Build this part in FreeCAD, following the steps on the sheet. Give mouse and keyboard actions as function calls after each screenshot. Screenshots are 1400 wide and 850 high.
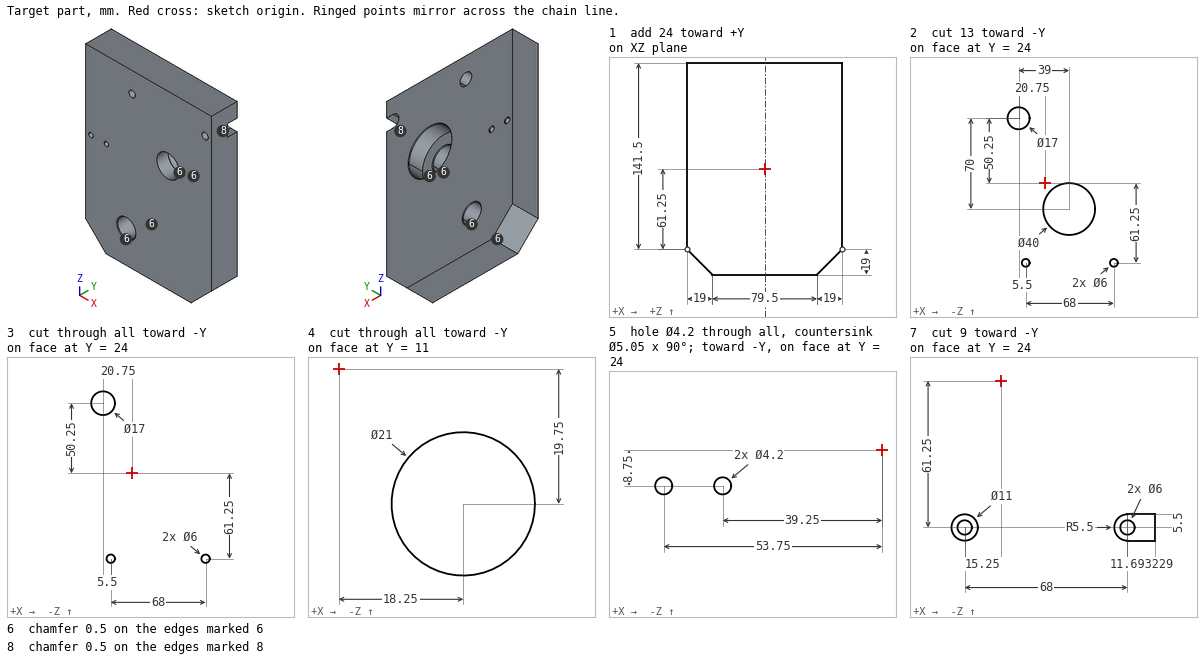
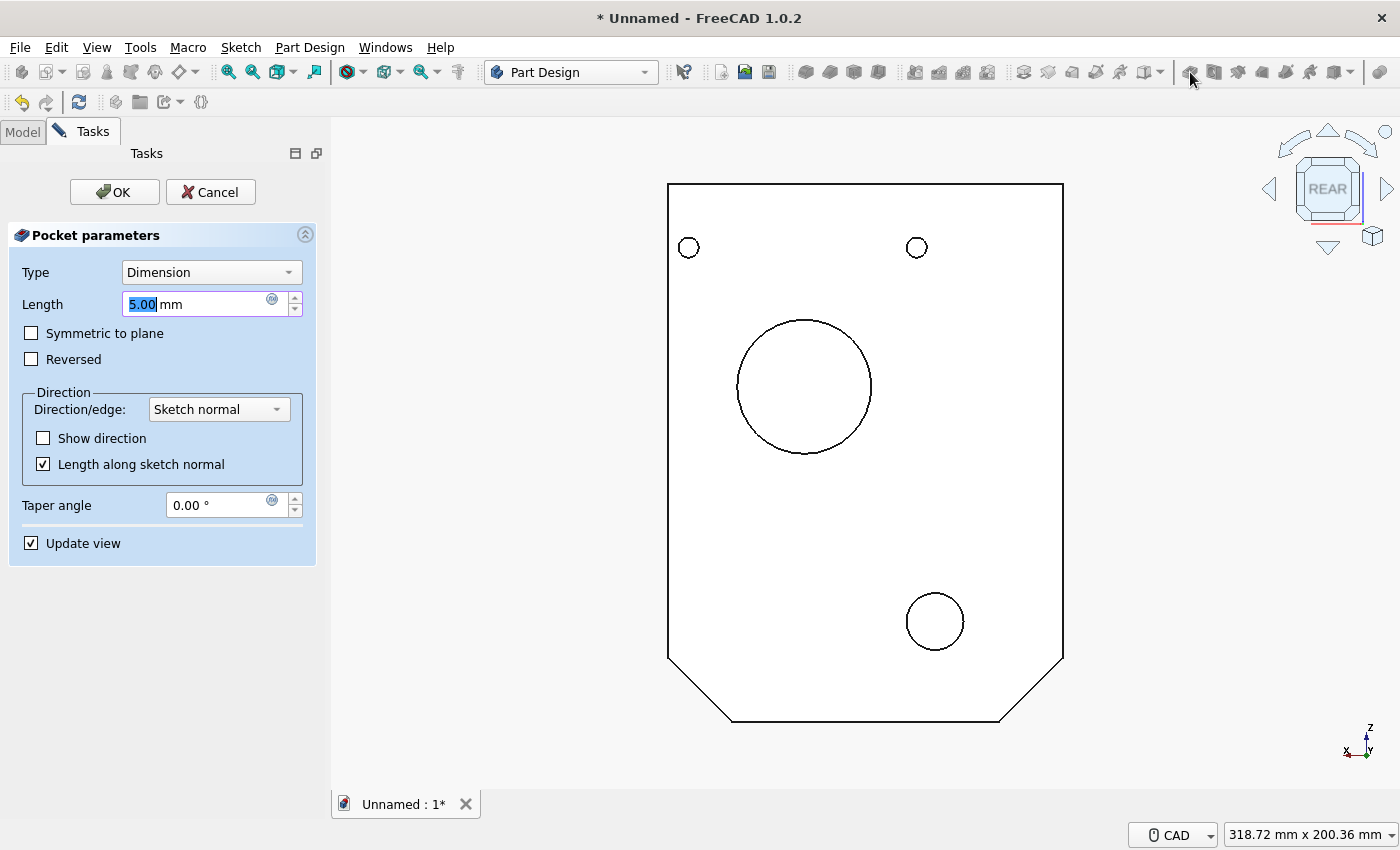
text(13)
key(Tab)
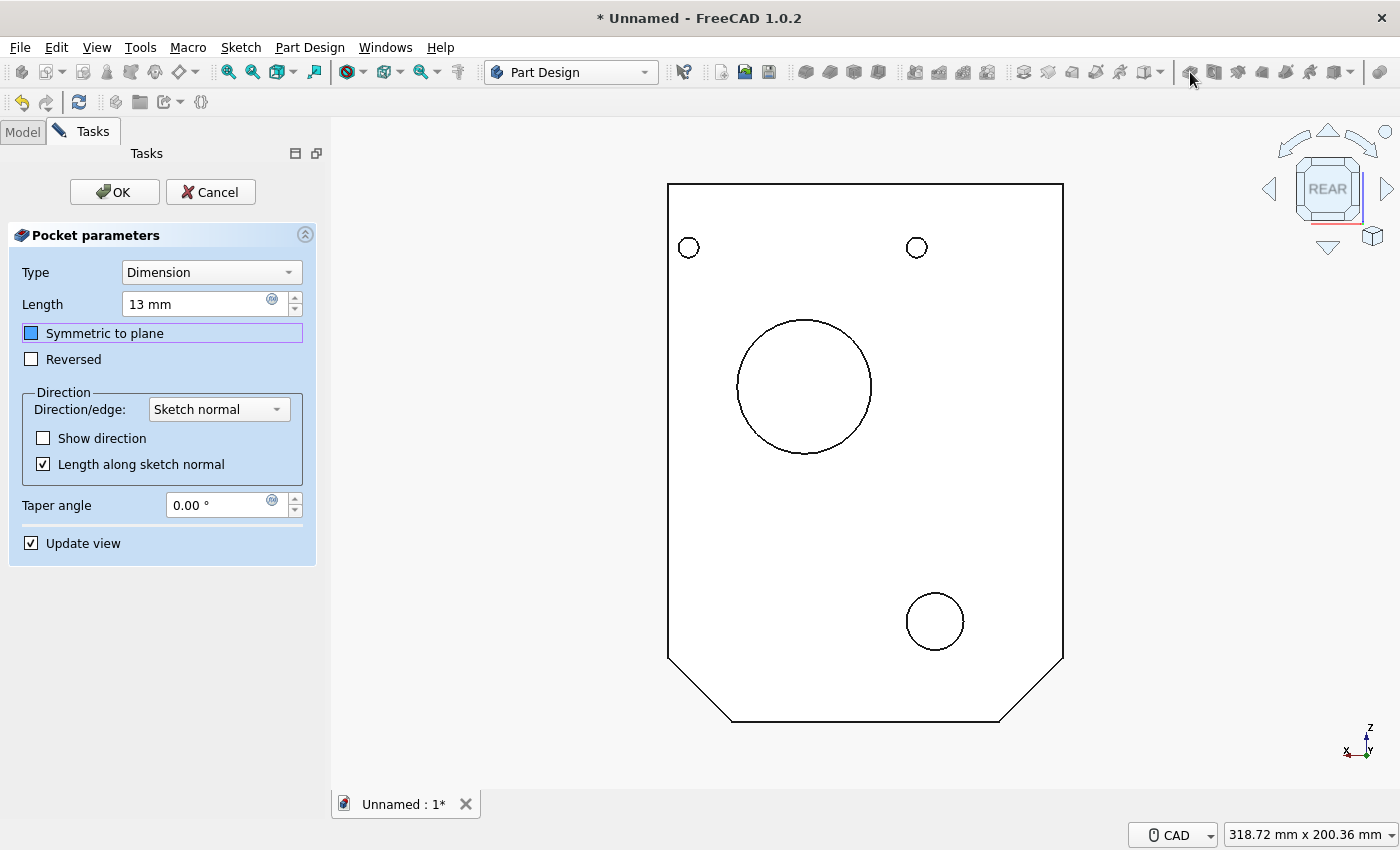
click(115, 192)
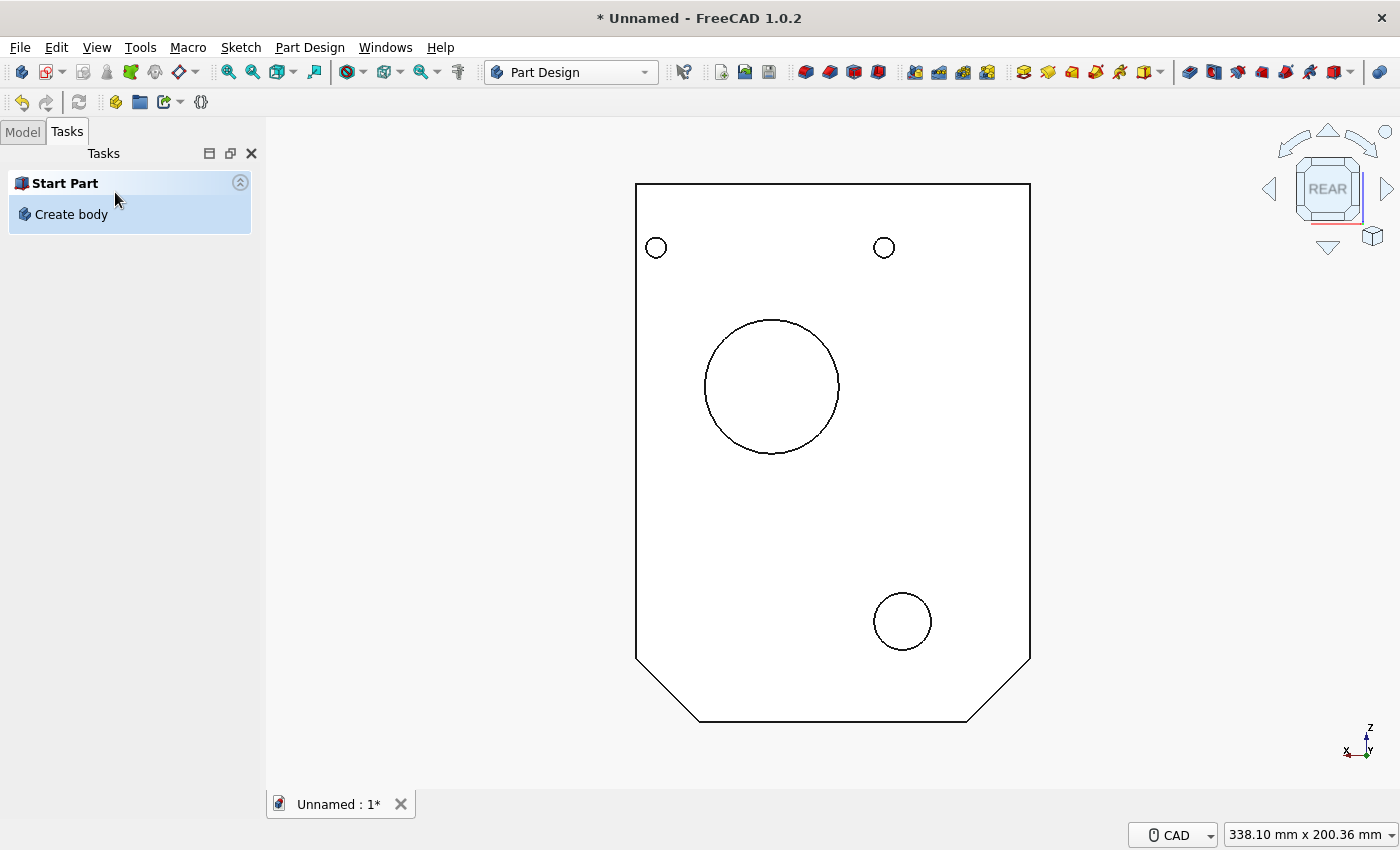
click(777, 606)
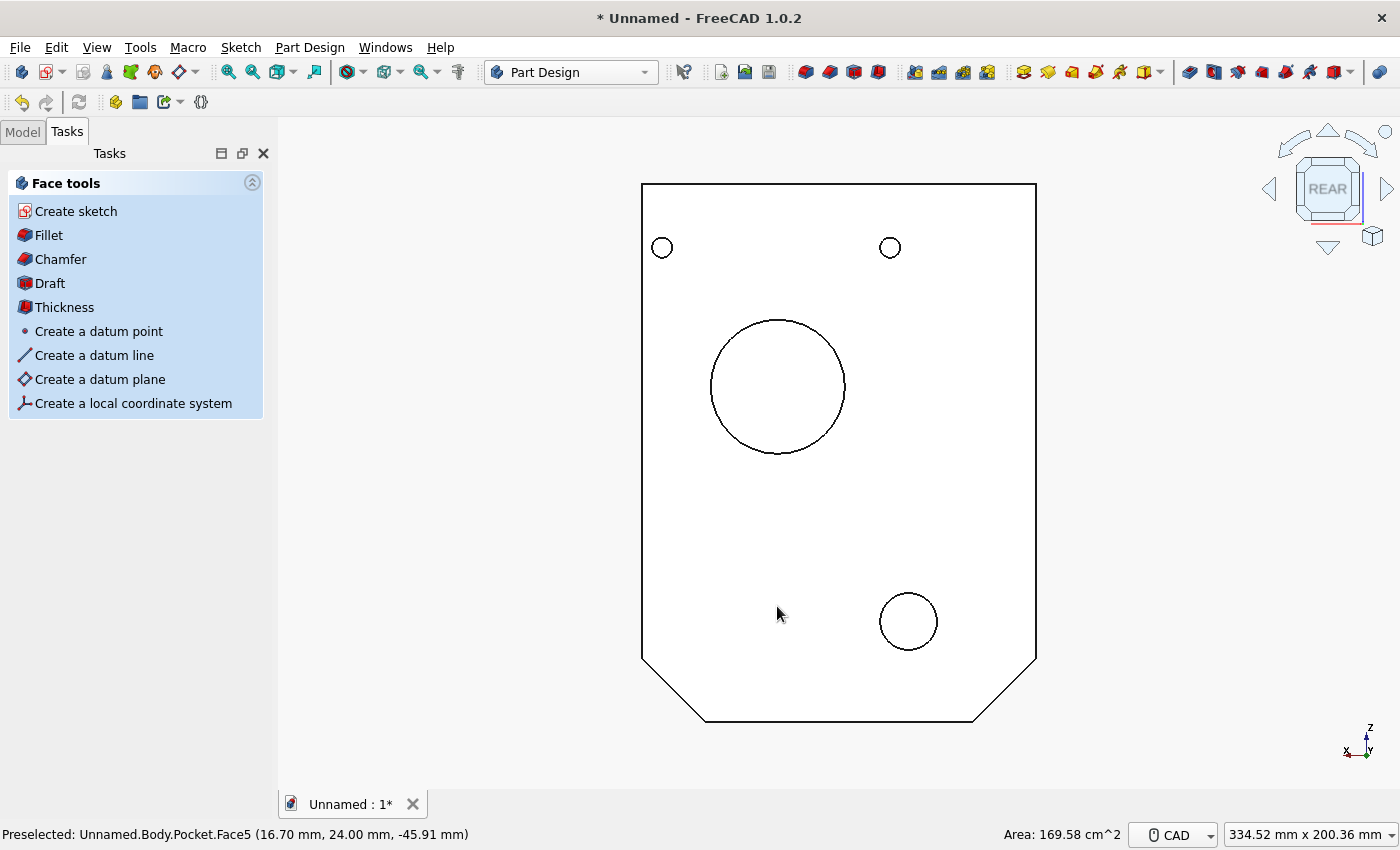
click(46, 72)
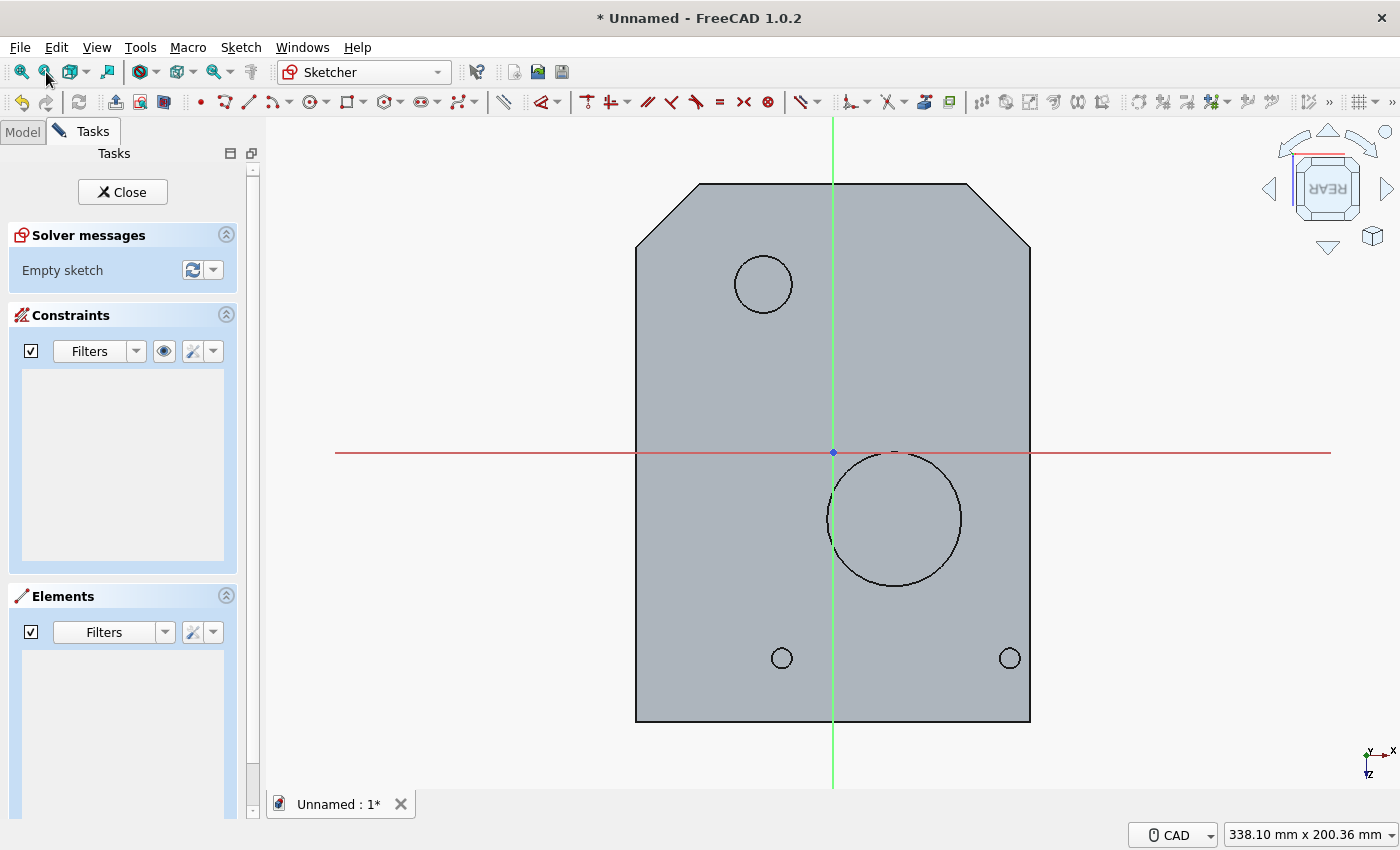
click(310, 102)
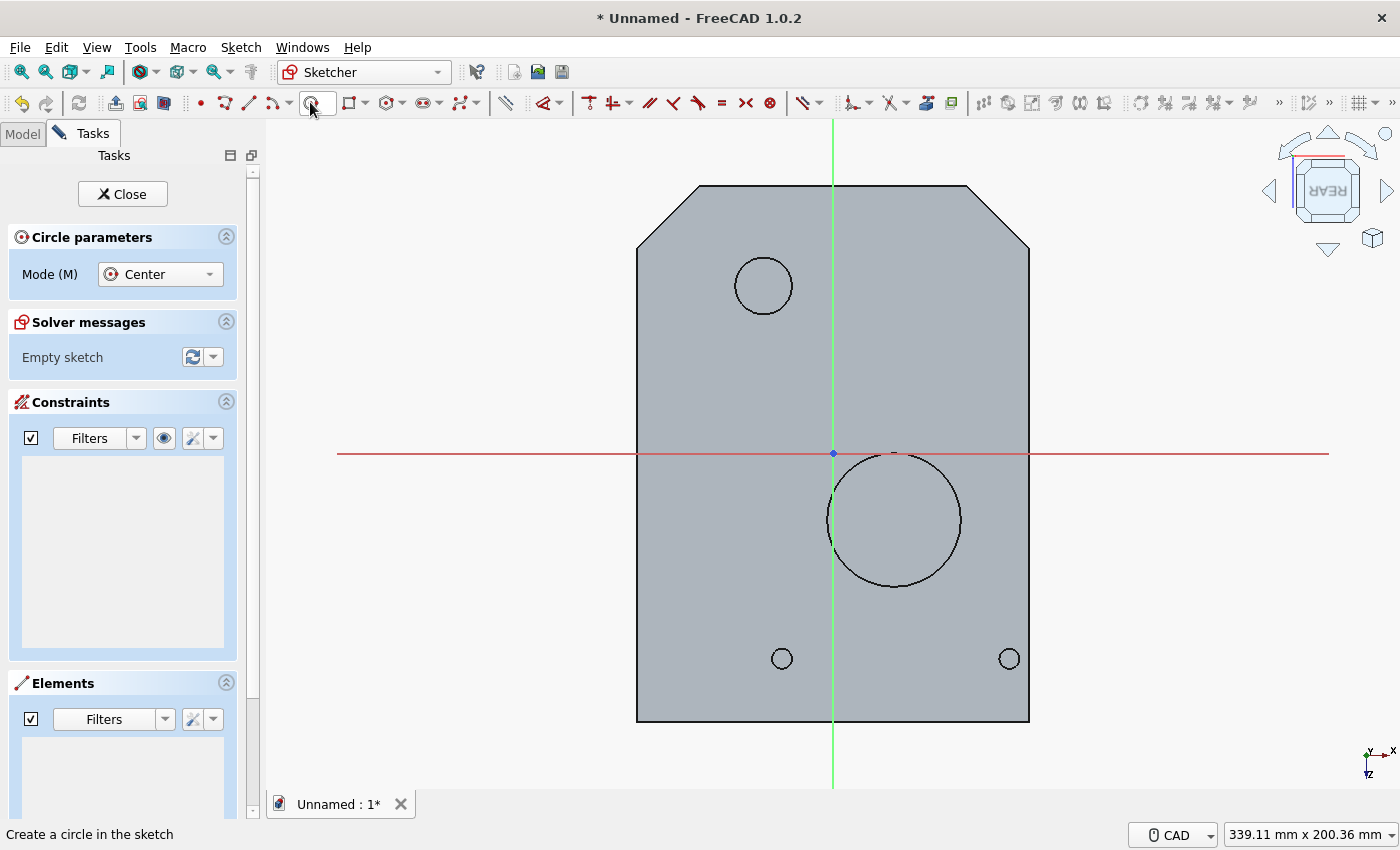
click(764, 286)
move(784, 266)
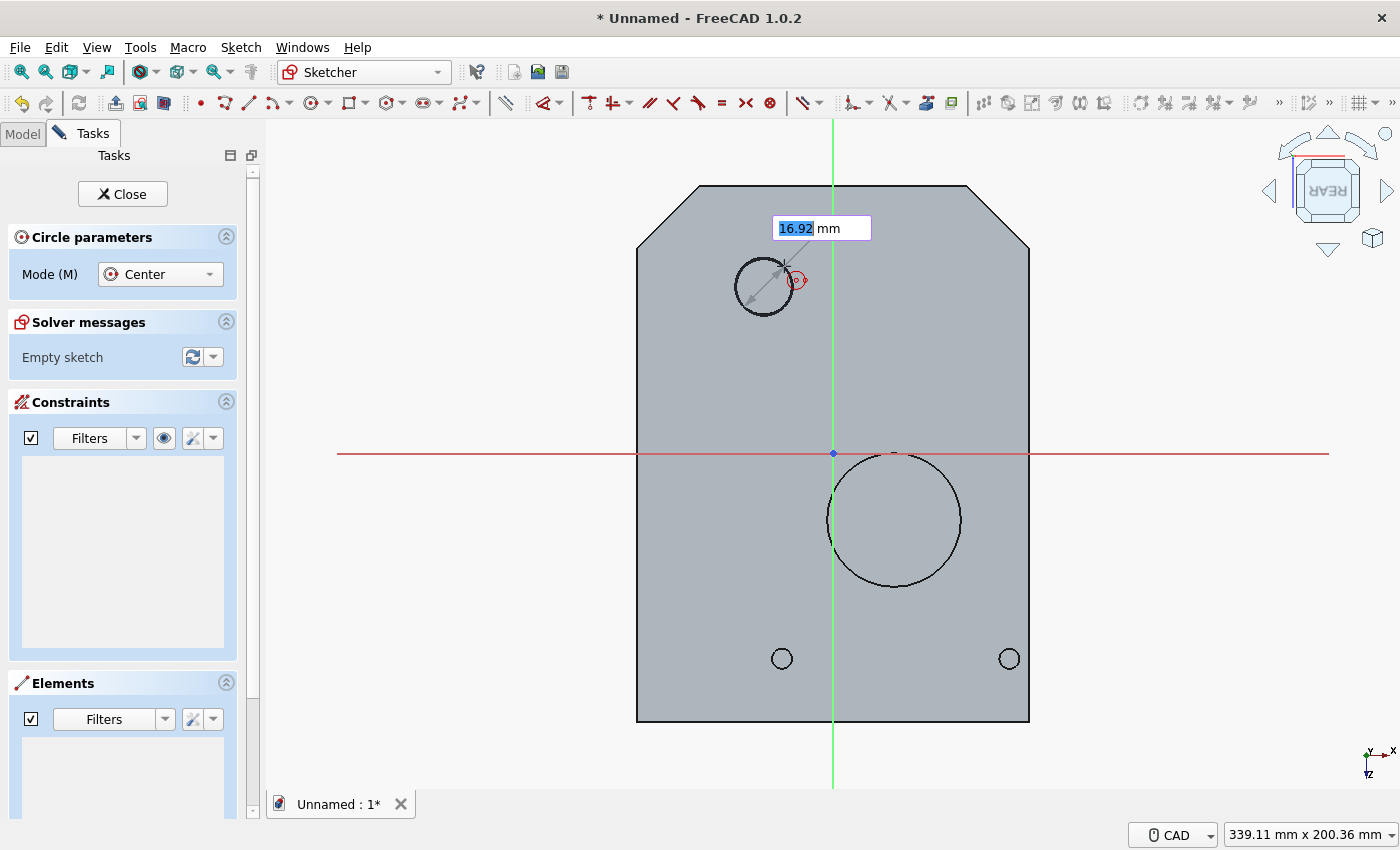
text(17)
key(Return)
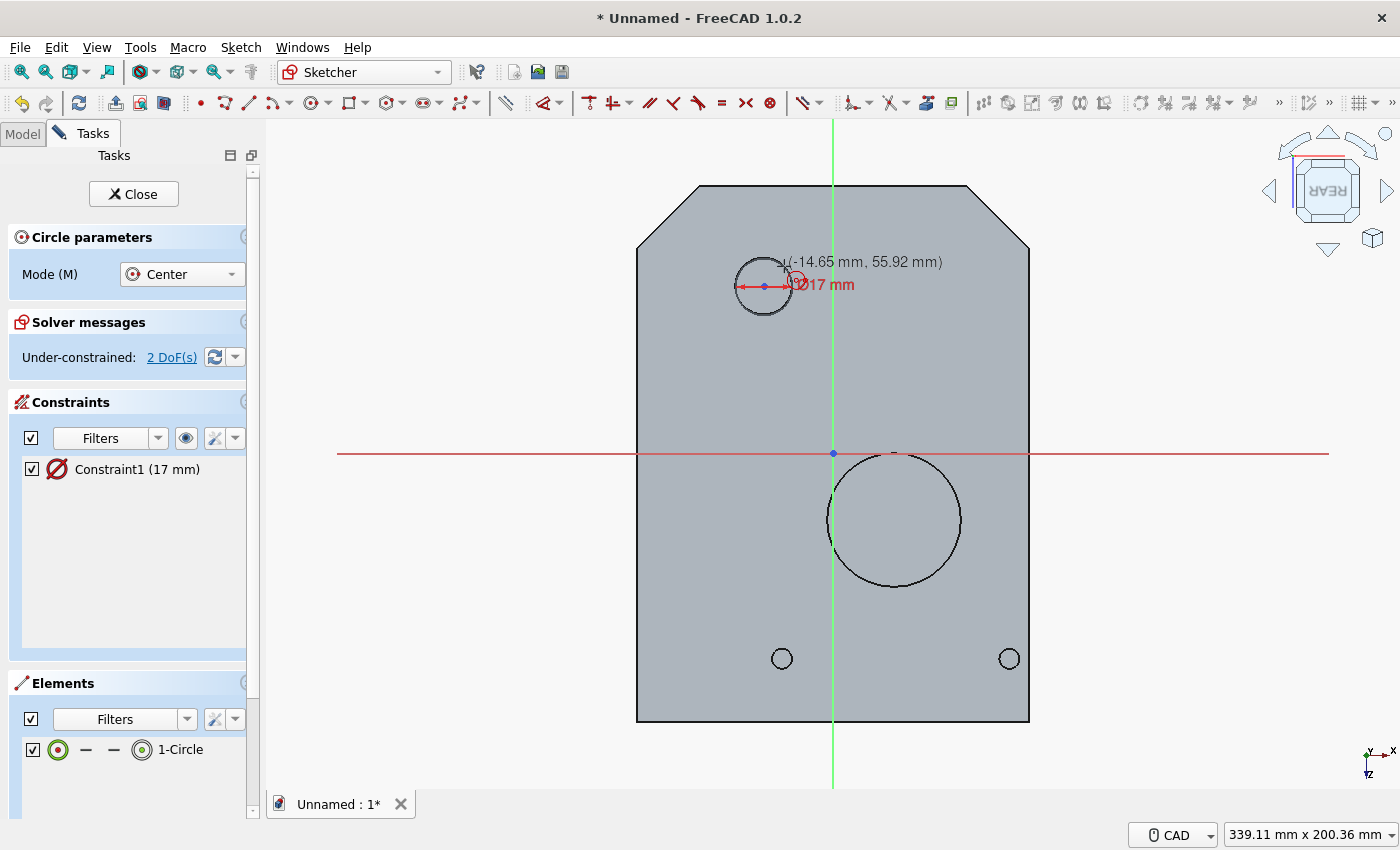
scroll(1009, 659, up, 5)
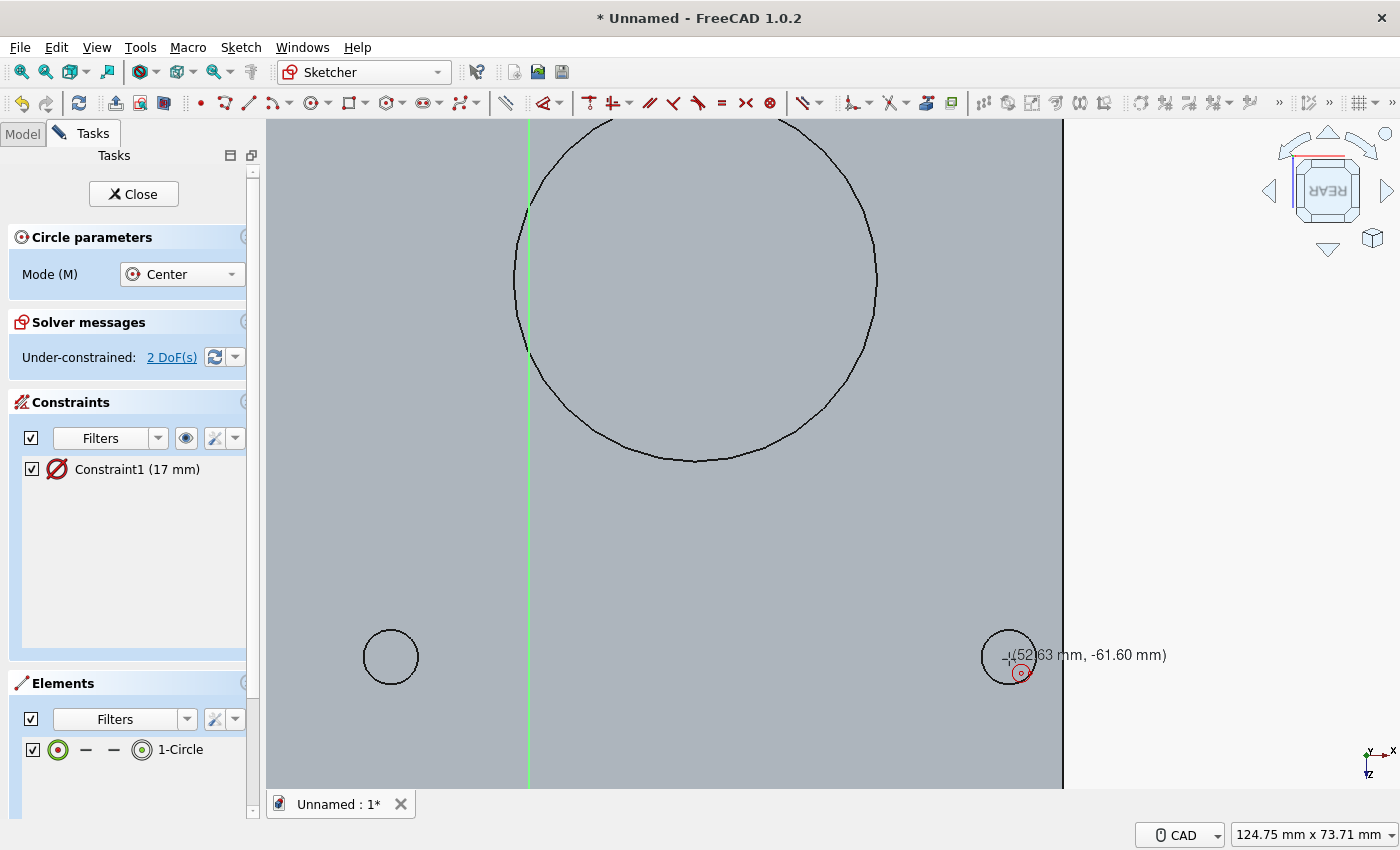
click(1009, 657)
move(1028, 638)